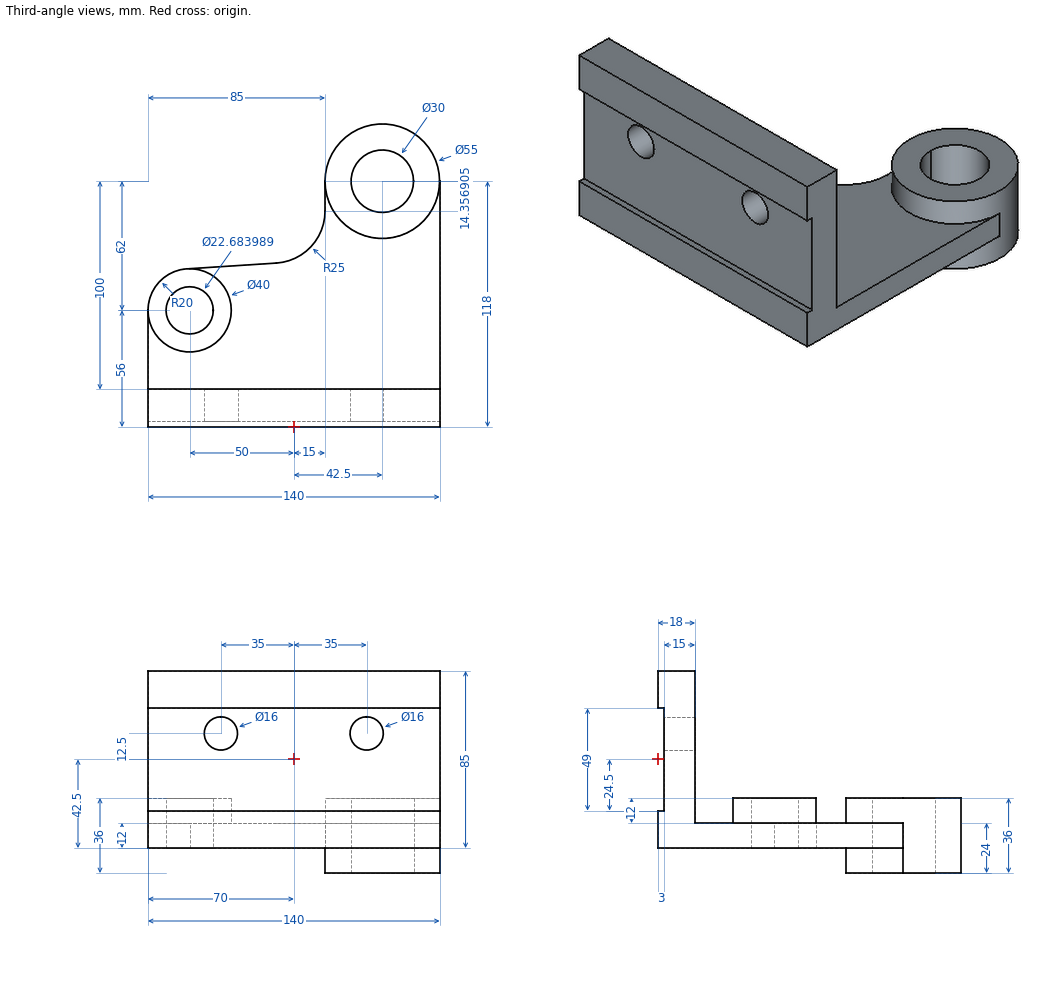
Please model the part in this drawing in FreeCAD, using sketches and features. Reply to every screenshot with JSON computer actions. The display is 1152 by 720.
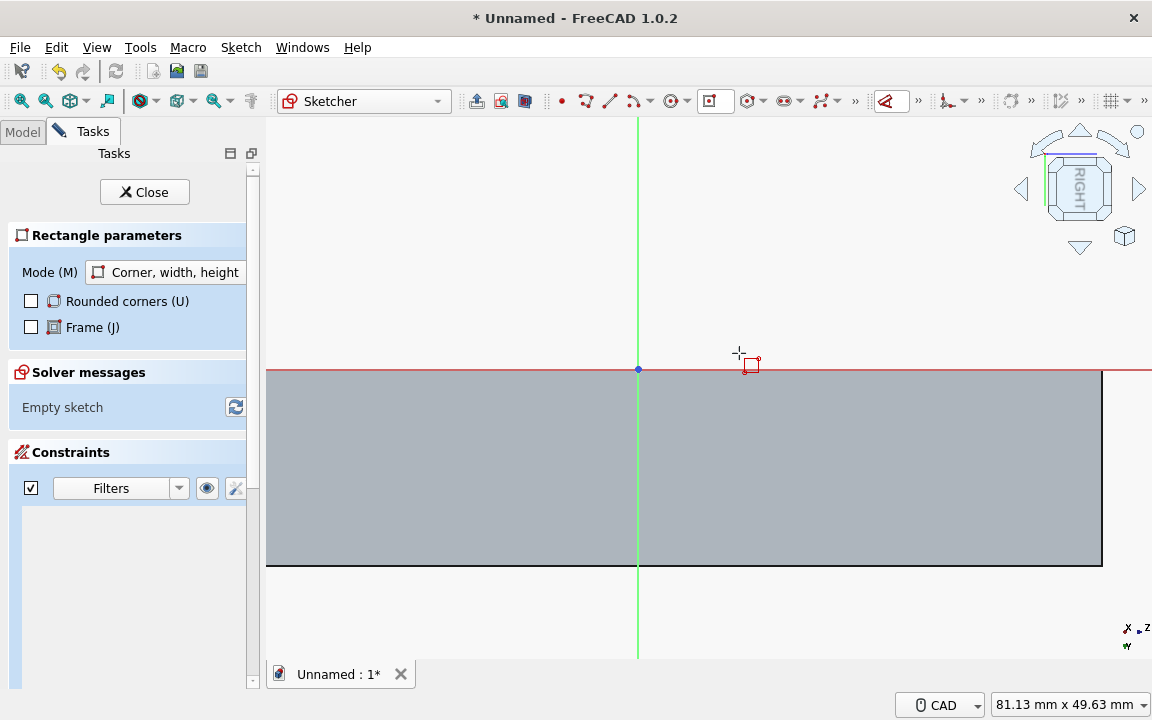
{"action": "left_click", "coordinate": [371, 370]}
{"action": "left_click", "coordinate": [906, 403]}
{"action": "key", "text": "Escape"}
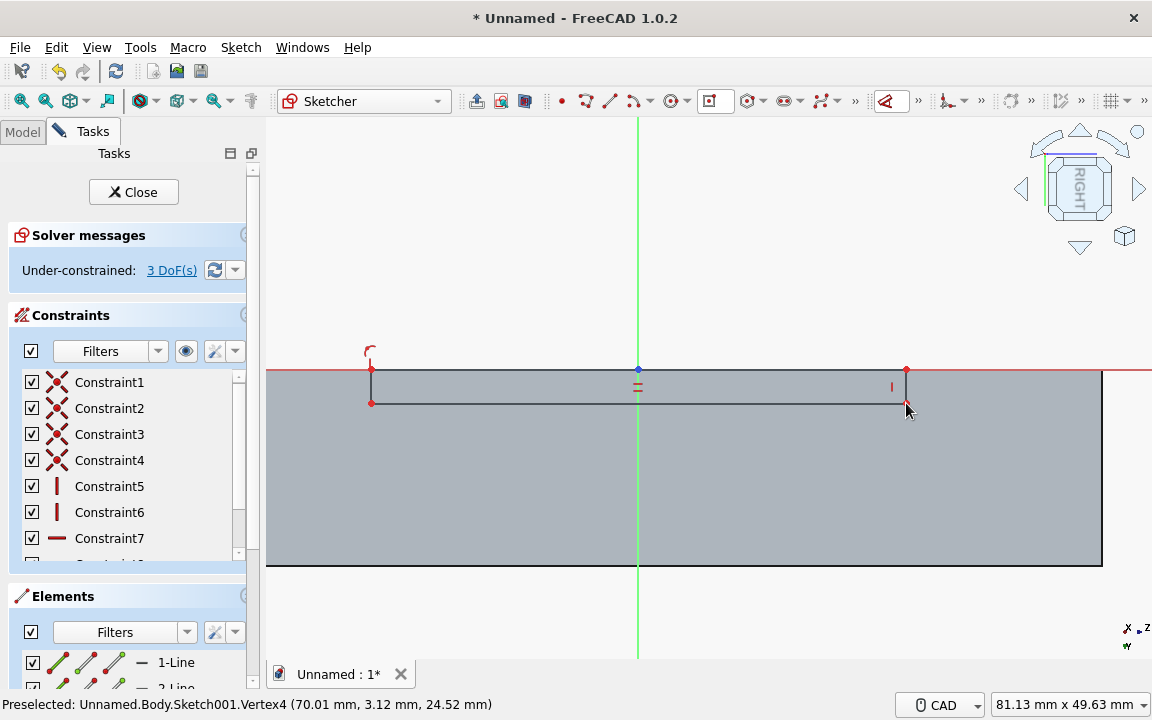
{"action": "scroll", "coordinate": [371, 380], "scroll_direction": "up", "scroll_amount": 2}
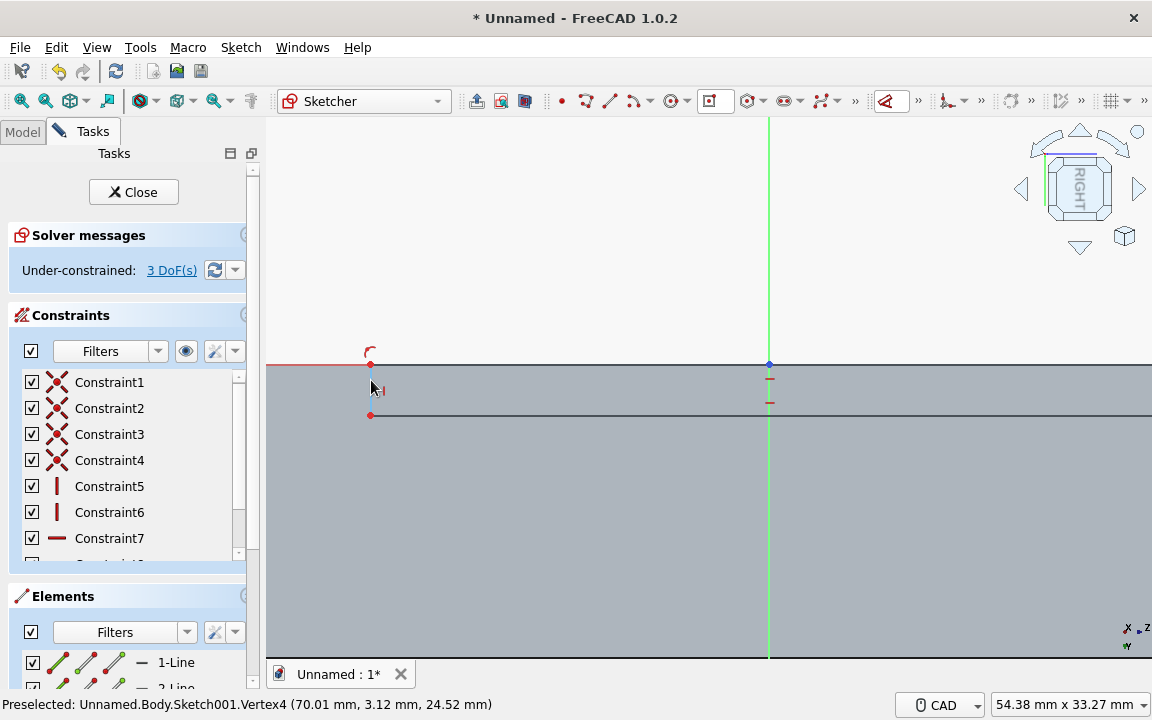
{"action": "left_click", "coordinate": [371, 380]}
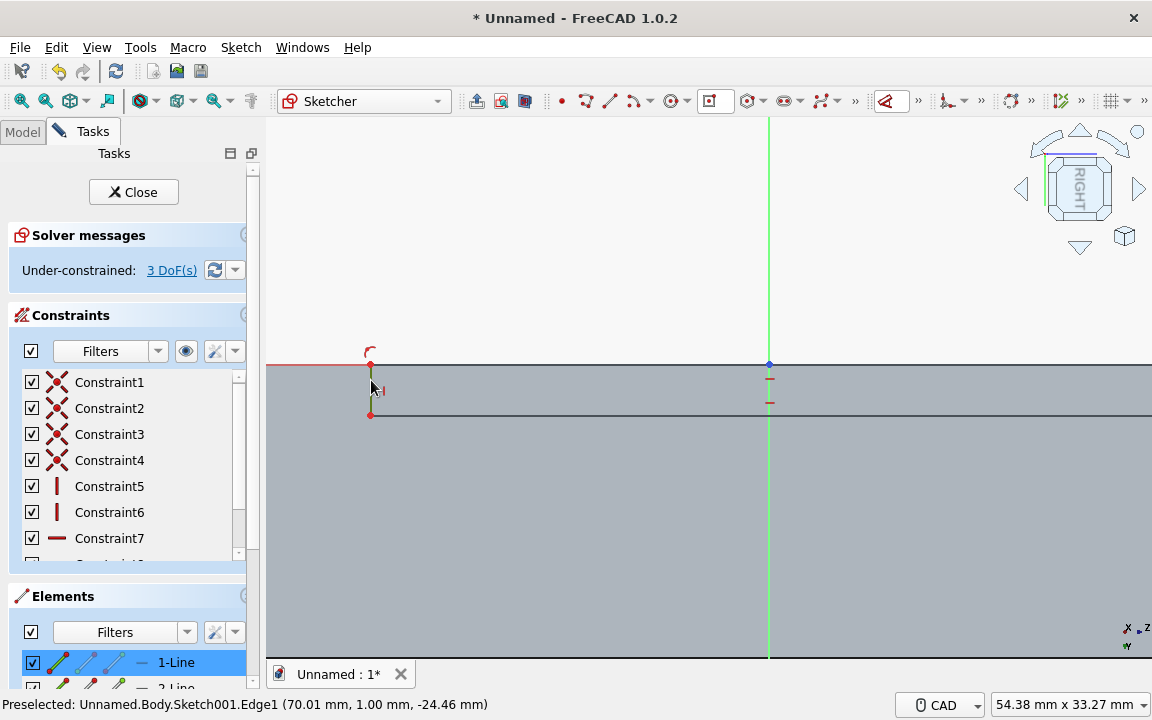
{"action": "key", "text": "i"}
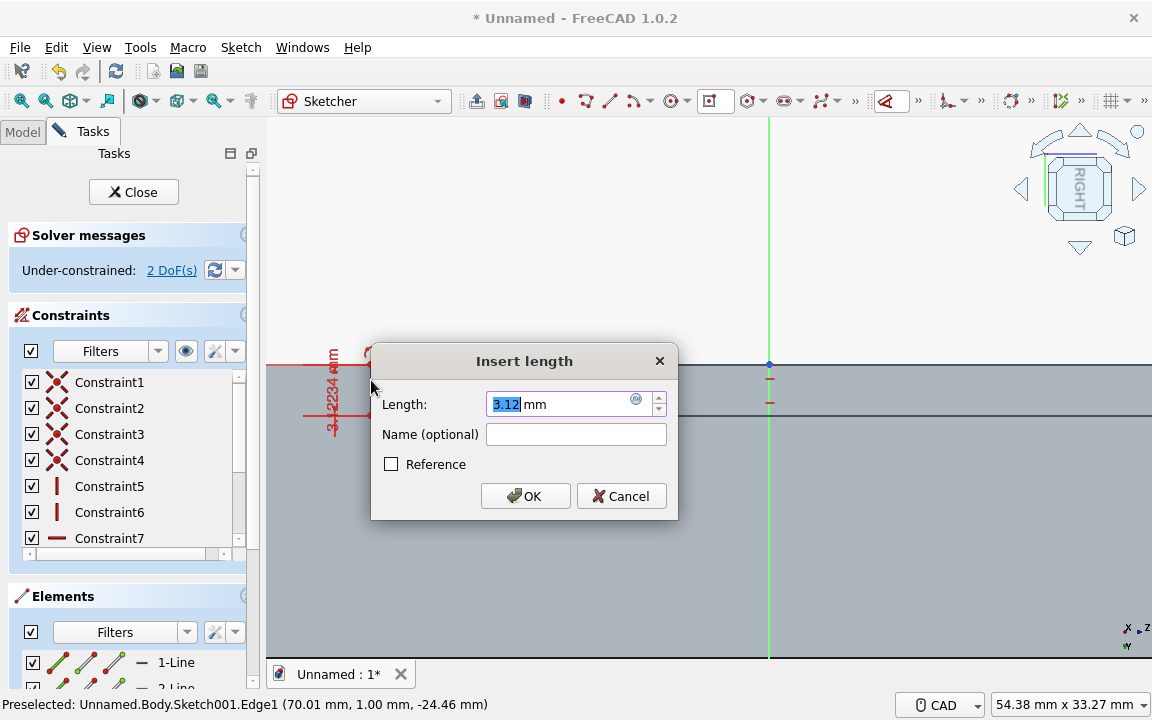
{"action": "type", "text": "3"}
{"action": "key", "text": "Return"}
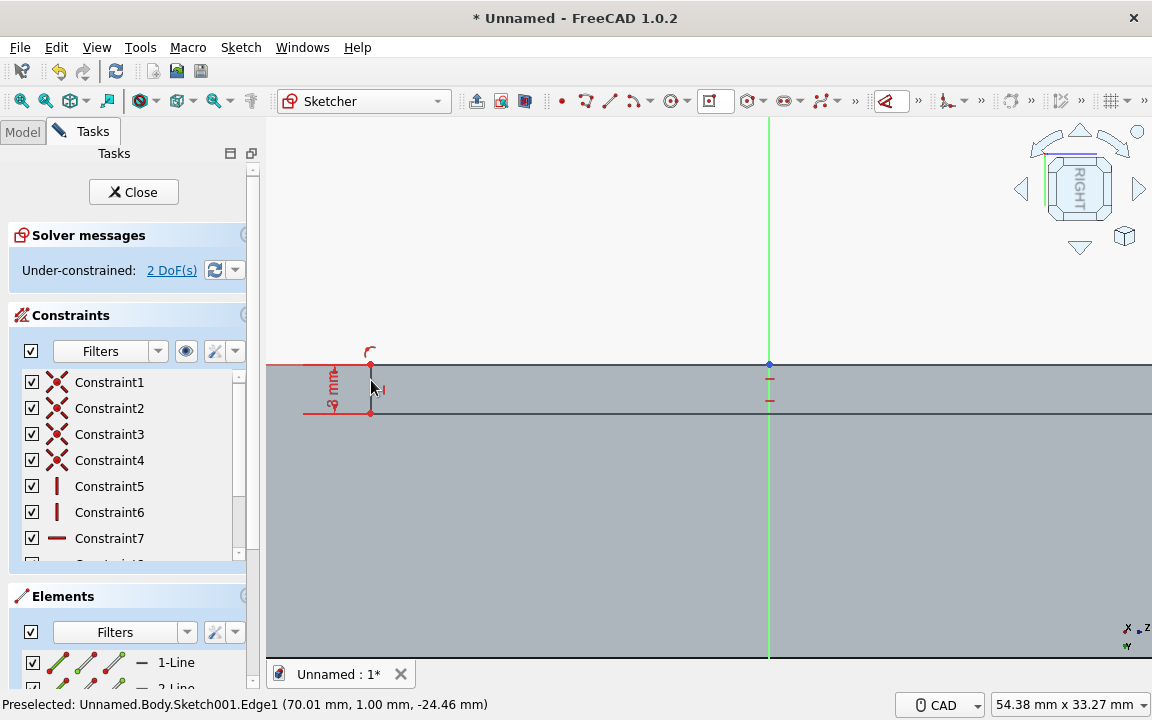
{"action": "left_click", "coordinate": [610, 414]}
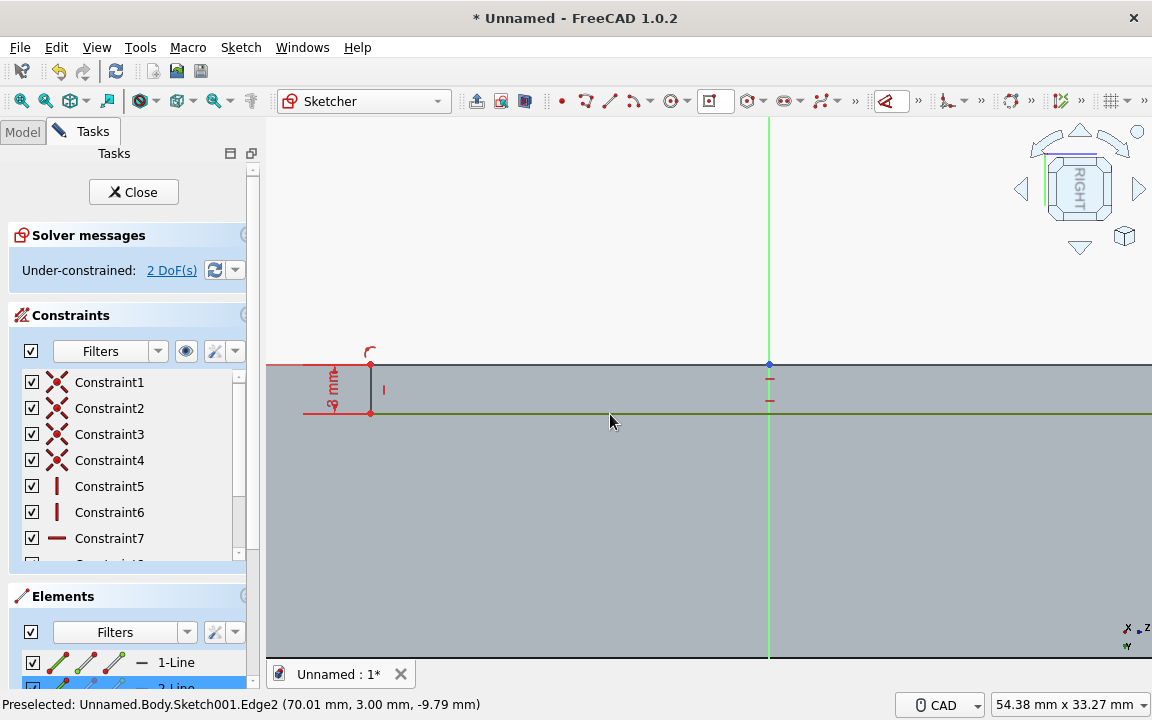
{"action": "key", "text": "l"}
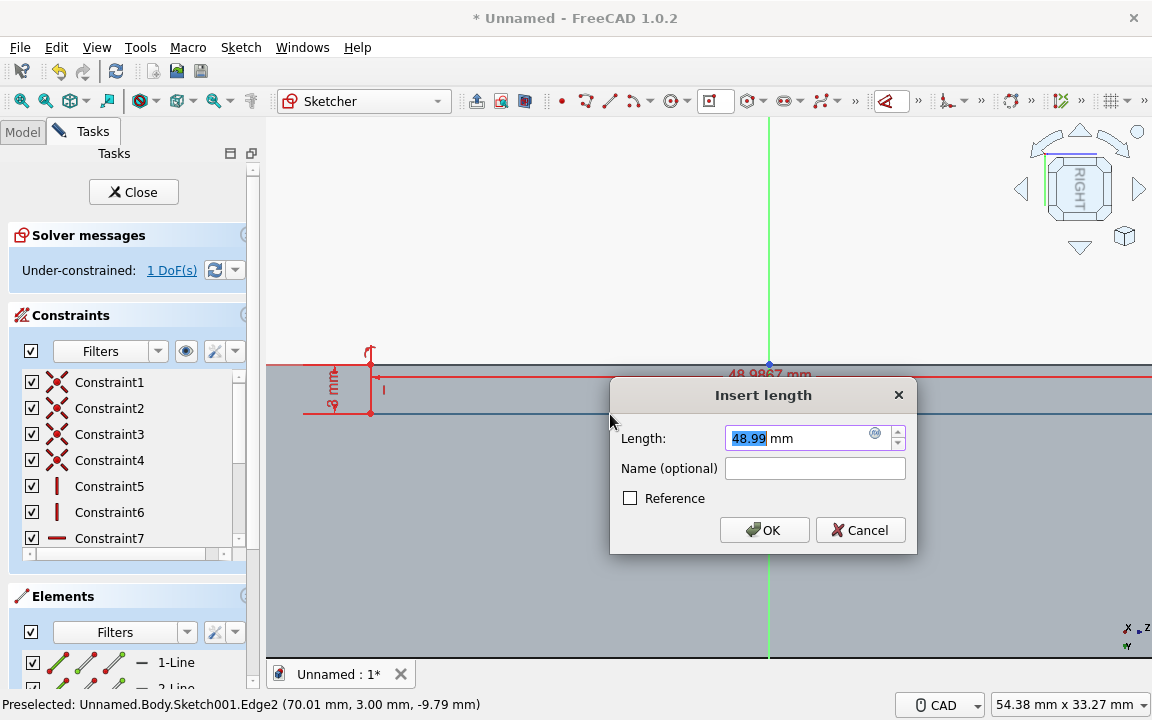
{"action": "type", "text": "49"}
{"action": "key", "text": "Return"}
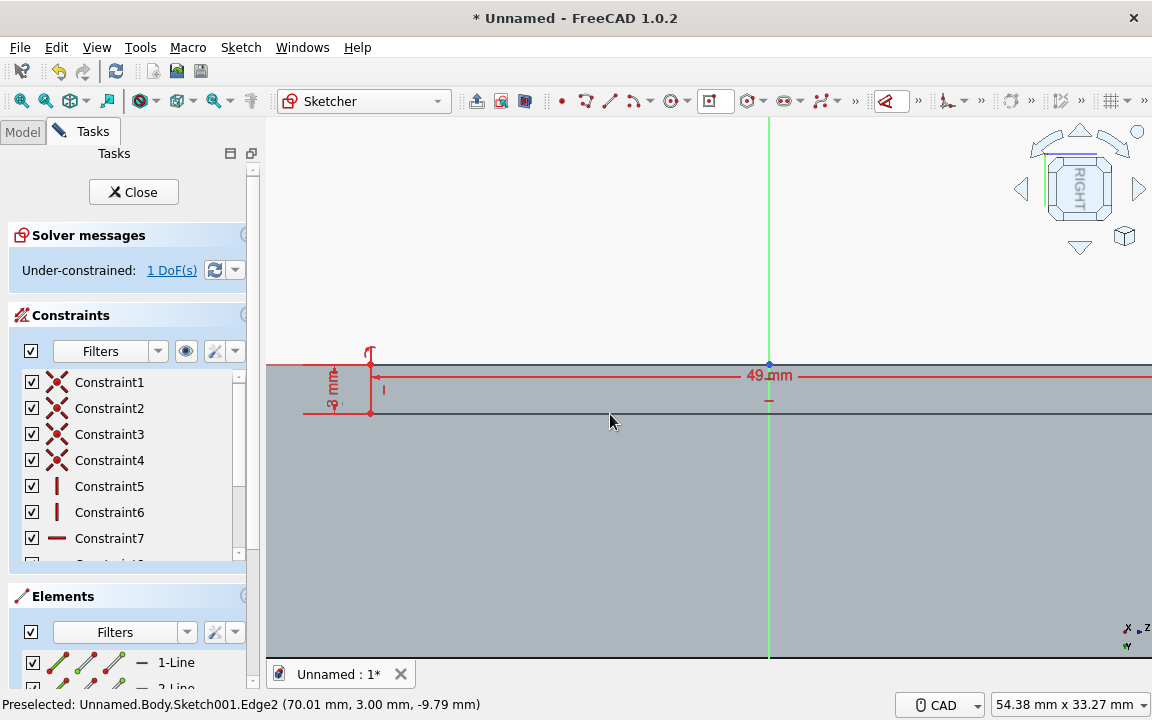
{"action": "left_click", "coordinate": [371, 365]}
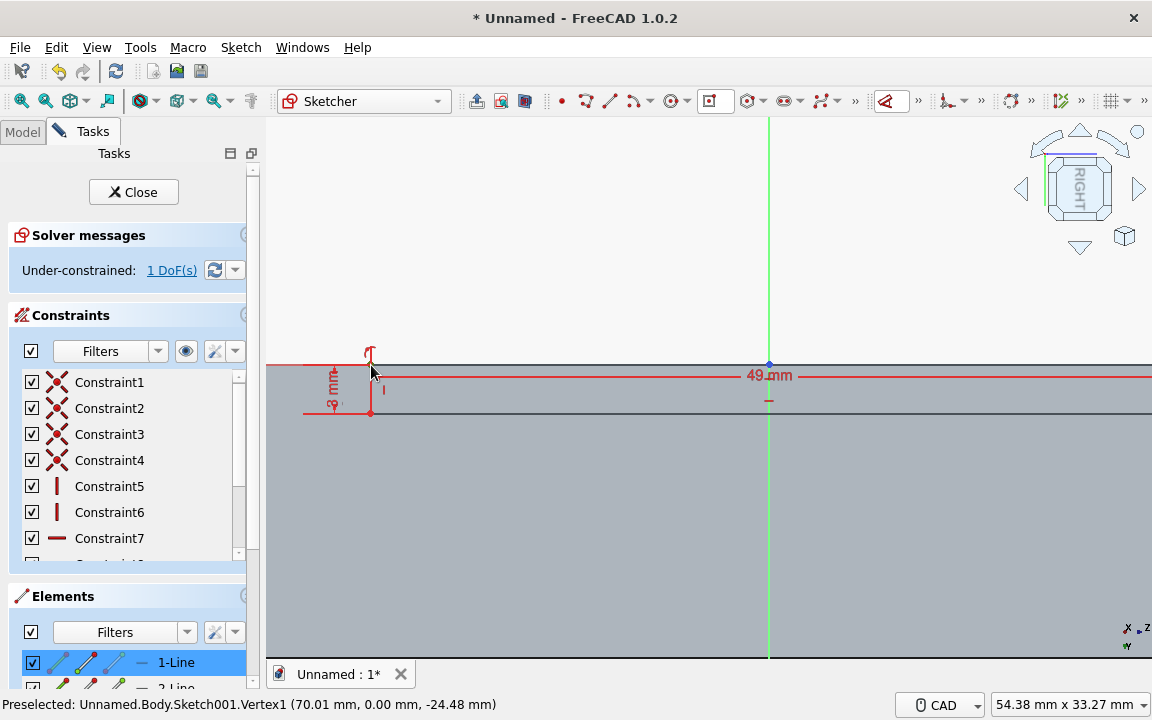
{"action": "key", "text": "l"}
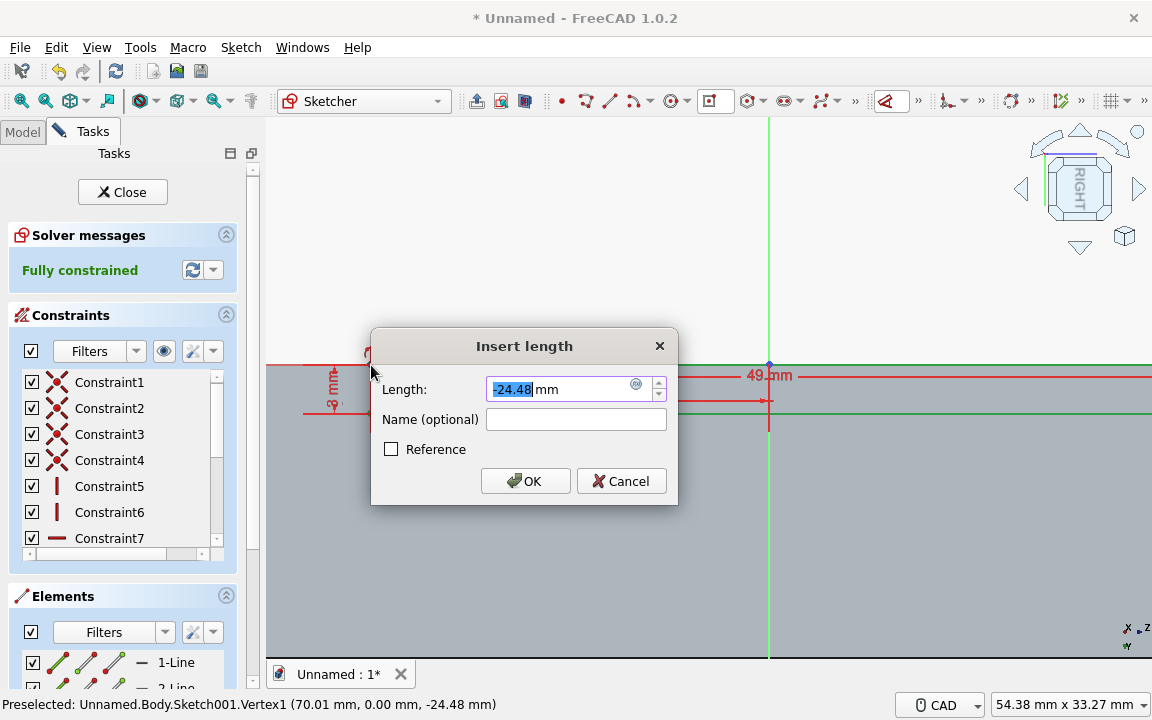
{"action": "type", "text": "-24.5"}
{"action": "key", "text": "Return"}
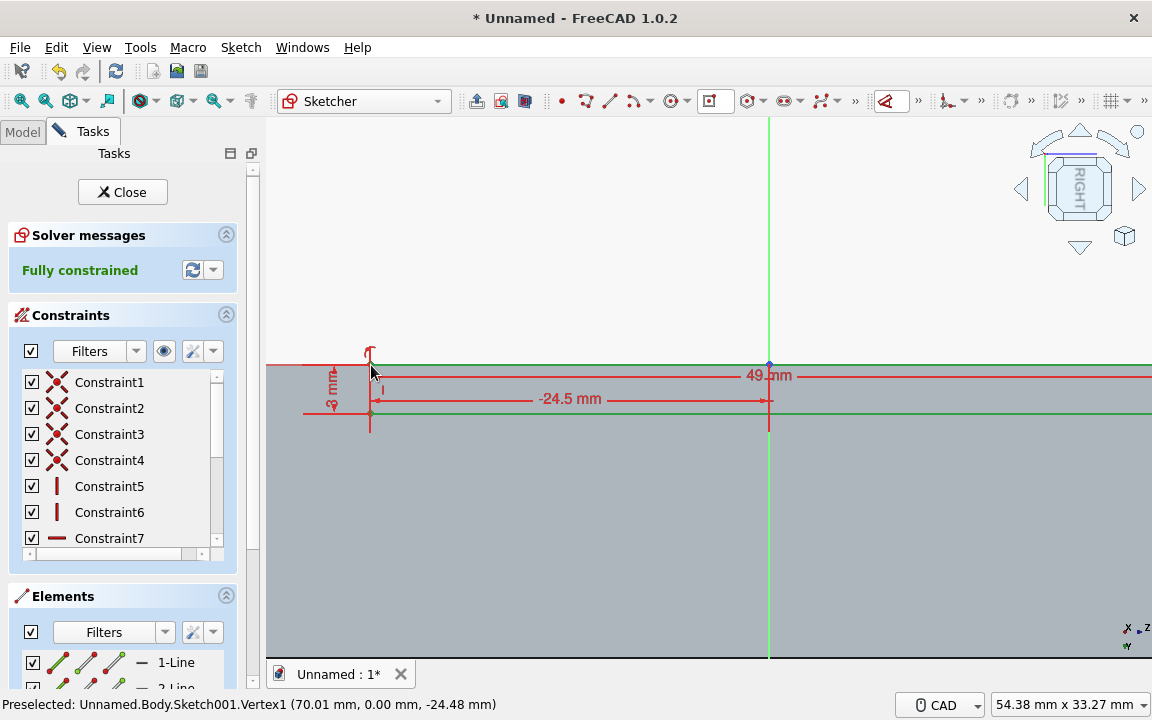
{"action": "left_click", "coordinate": [123, 192]}